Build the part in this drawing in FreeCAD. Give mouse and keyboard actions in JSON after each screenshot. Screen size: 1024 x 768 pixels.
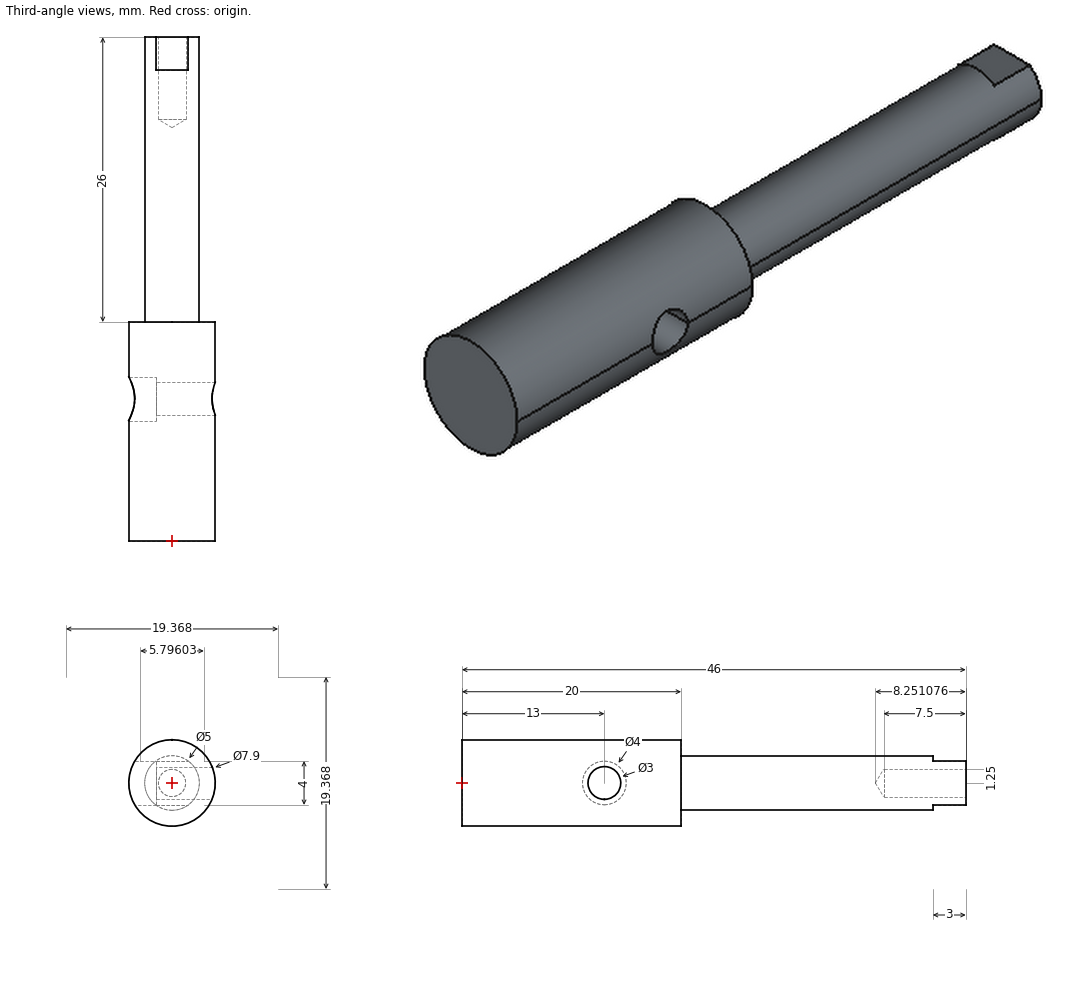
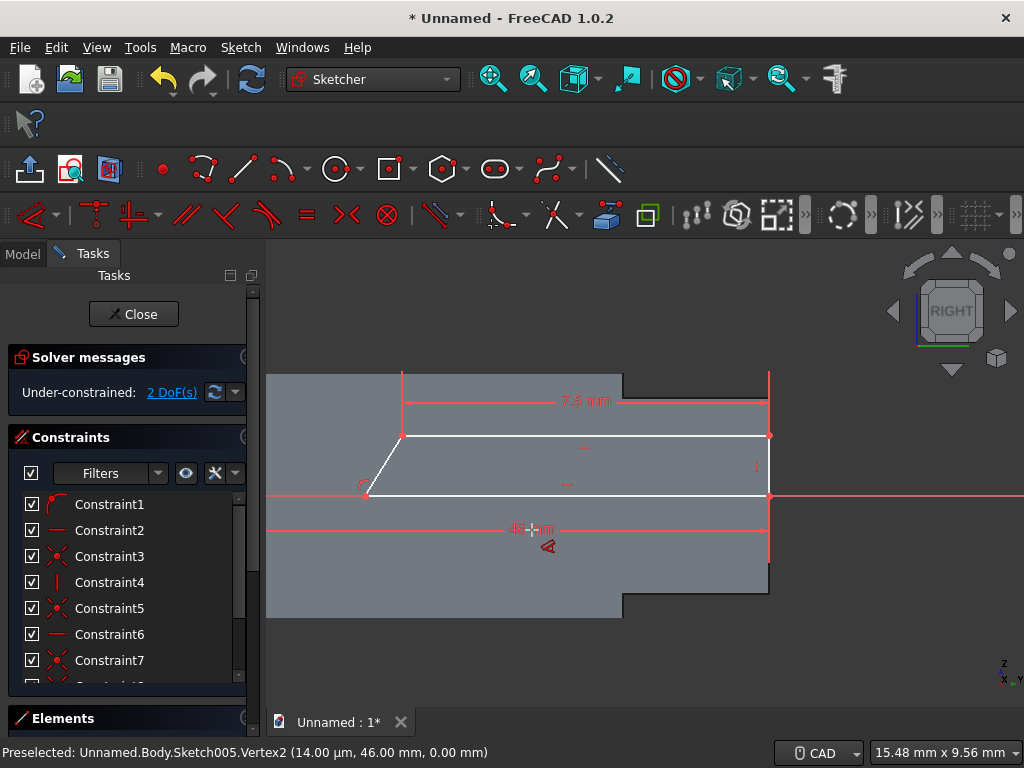
{"action": "left_click", "coordinate": [769, 478]}
{"action": "left_click", "coordinate": [803, 466]}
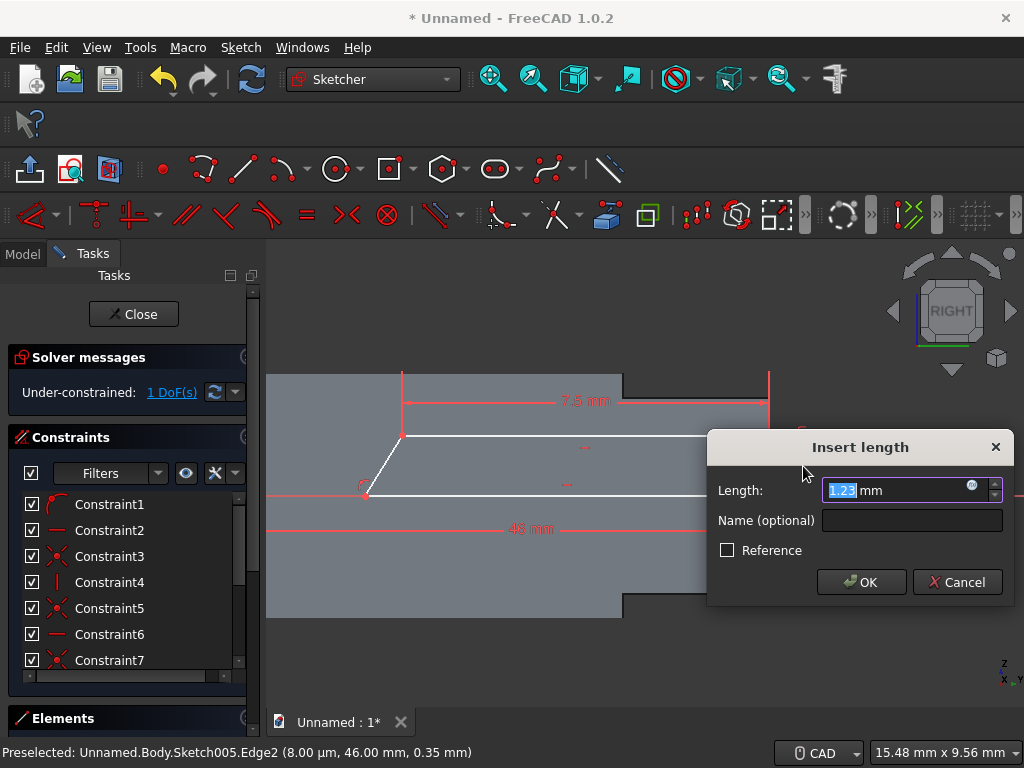
{"action": "type", "text": "1.25"}
{"action": "key", "text": "Return"}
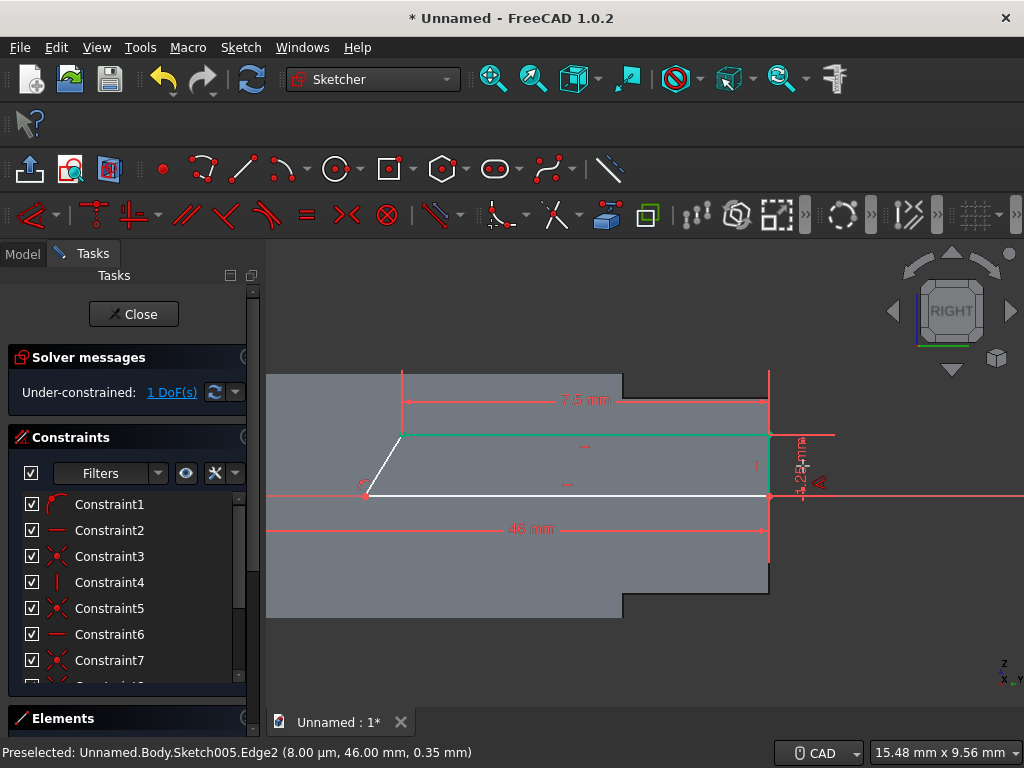
{"action": "left_click", "coordinate": [486, 496]}
{"action": "left_click", "coordinate": [660, 530]}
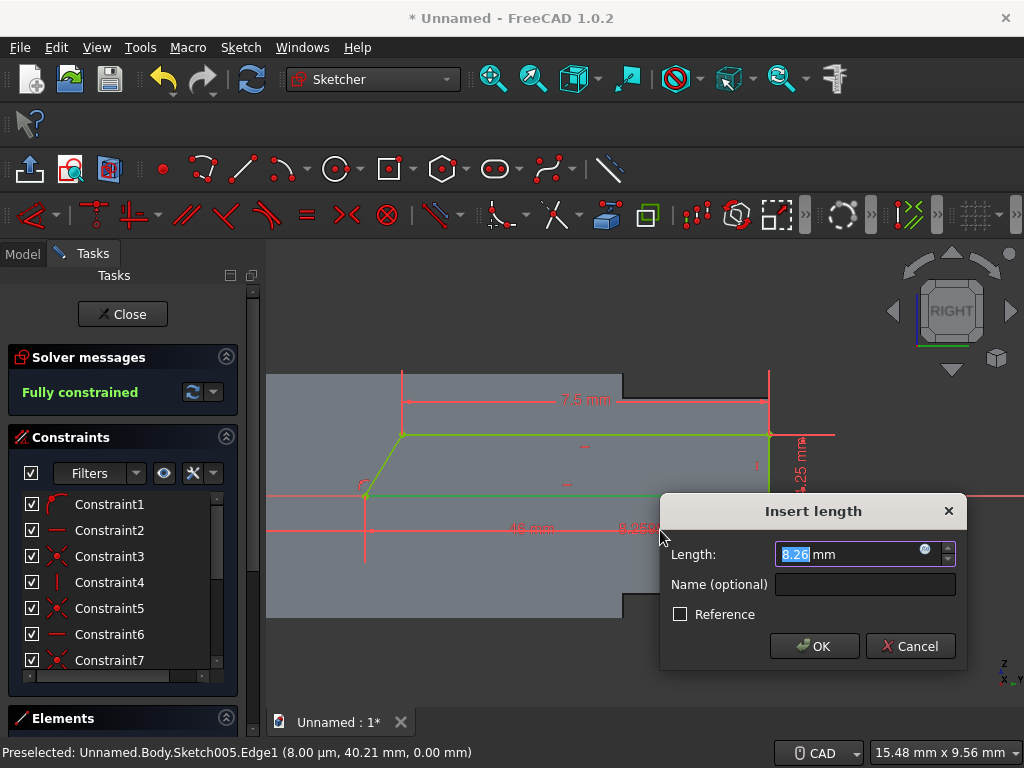
{"action": "type", "text": "8.251076"}
{"action": "key", "text": "Return"}
{"action": "key", "text": "Escape"}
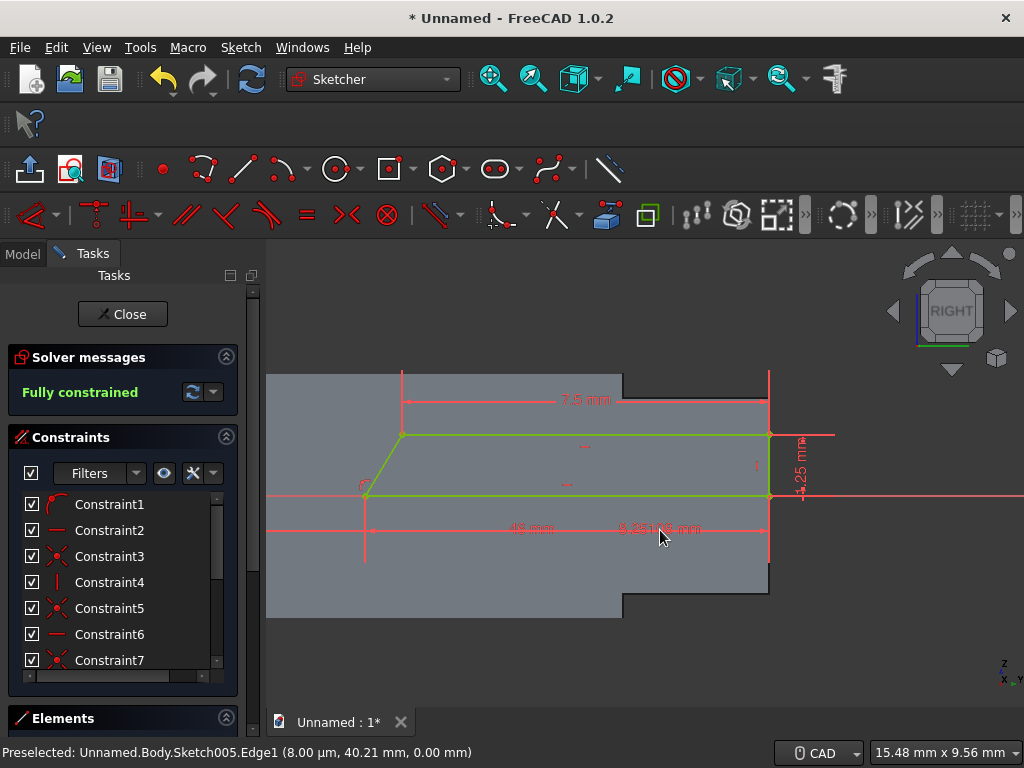
{"action": "left_click", "coordinate": [123, 314]}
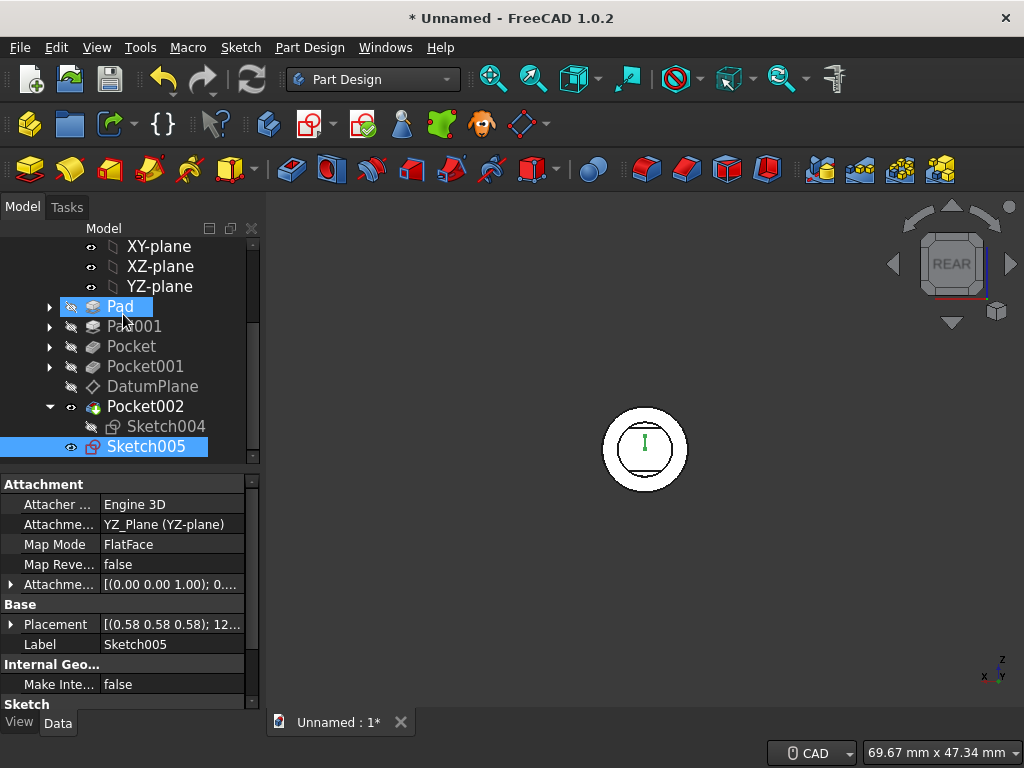
{"action": "left_click", "coordinate": [372, 170]}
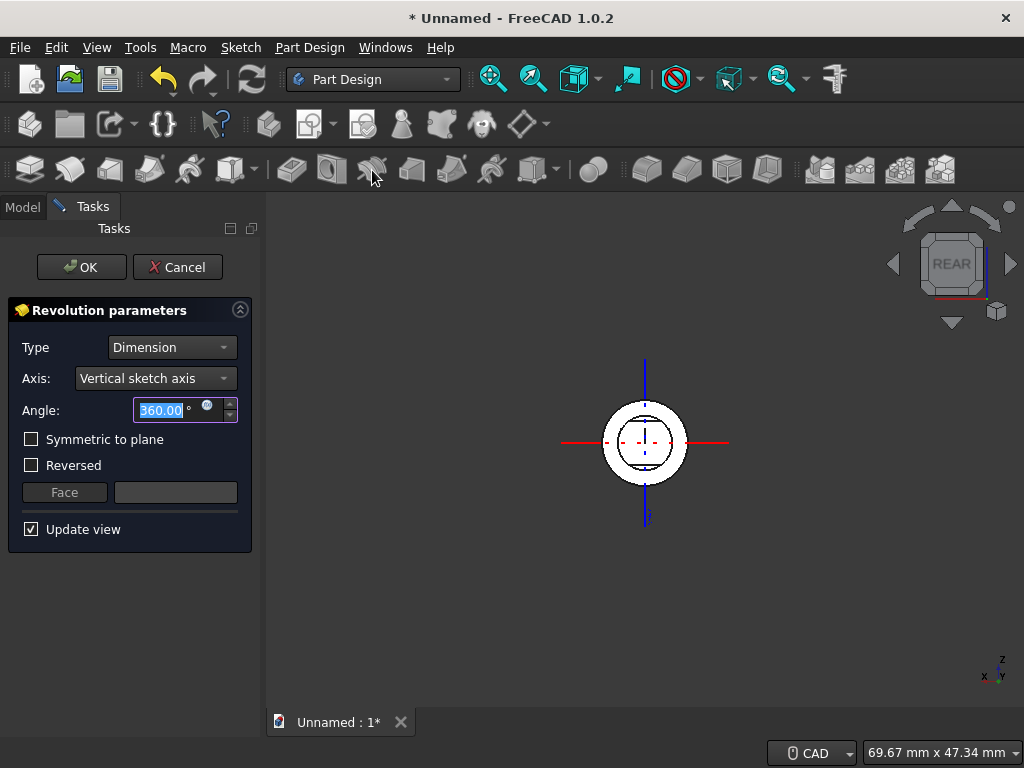
{"action": "left_click", "coordinate": [156, 378]}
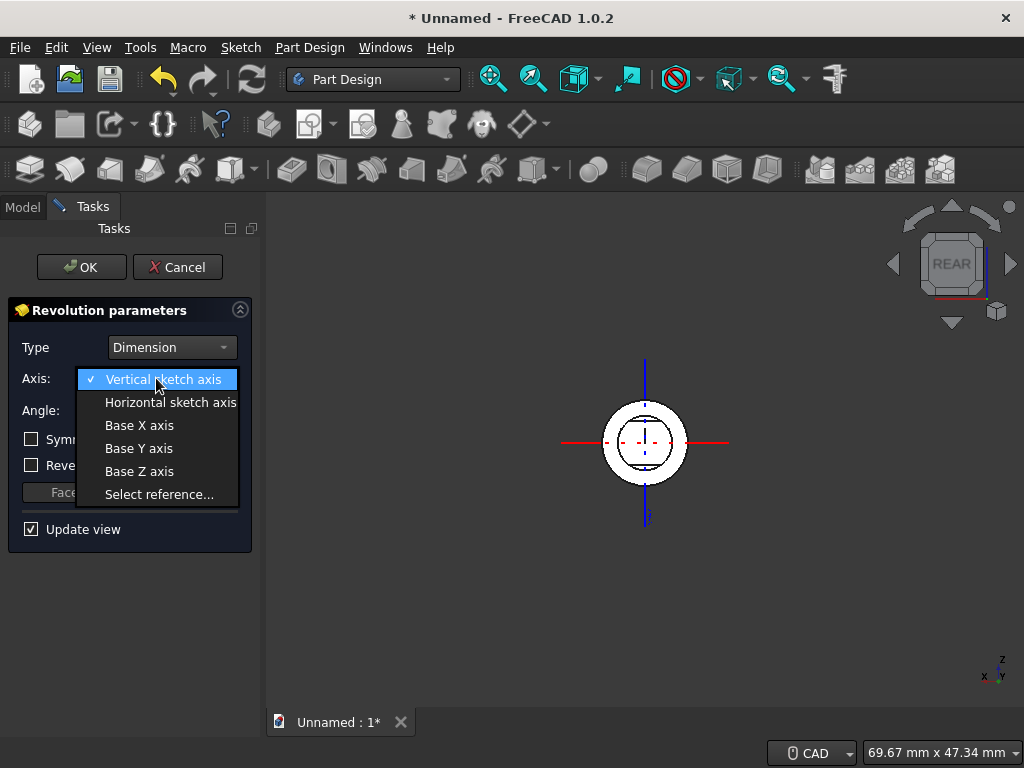
{"action": "left_click", "coordinate": [156, 402]}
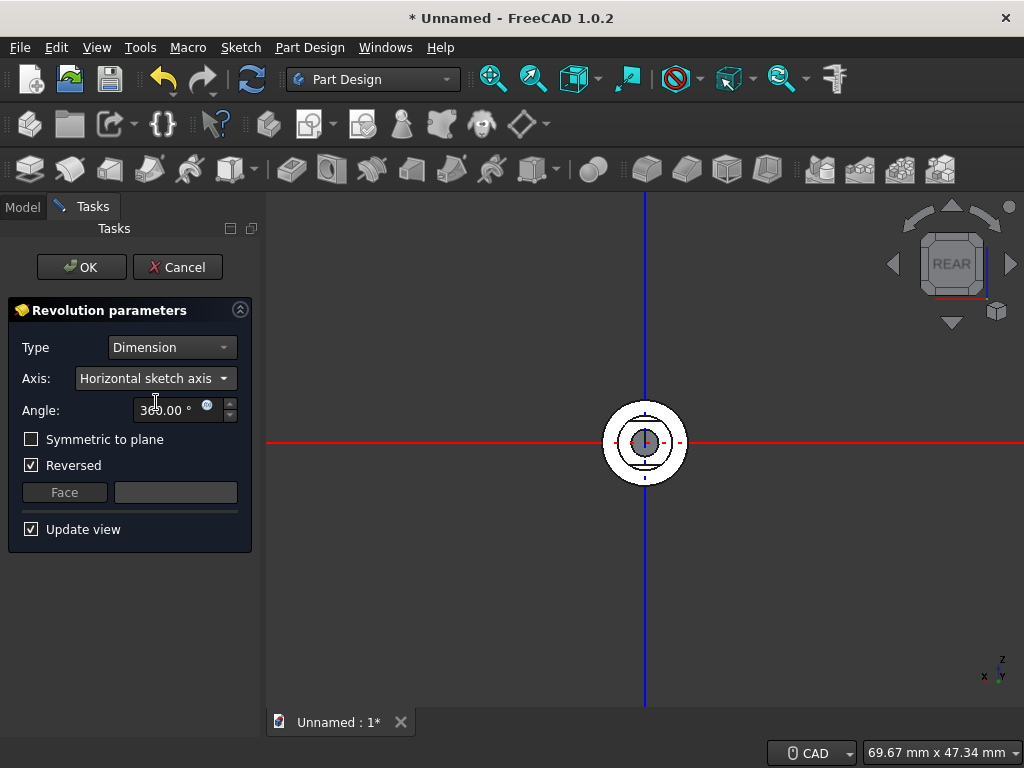
{"action": "left_click", "coordinate": [82, 267]}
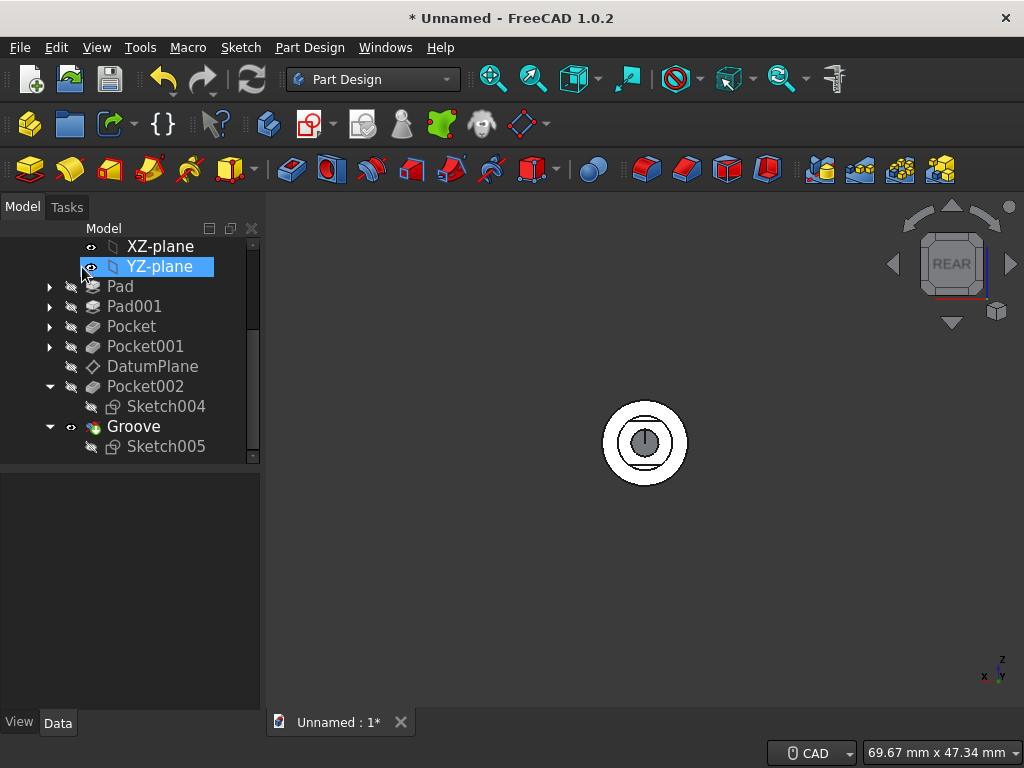
{"action": "key", "text": "0"}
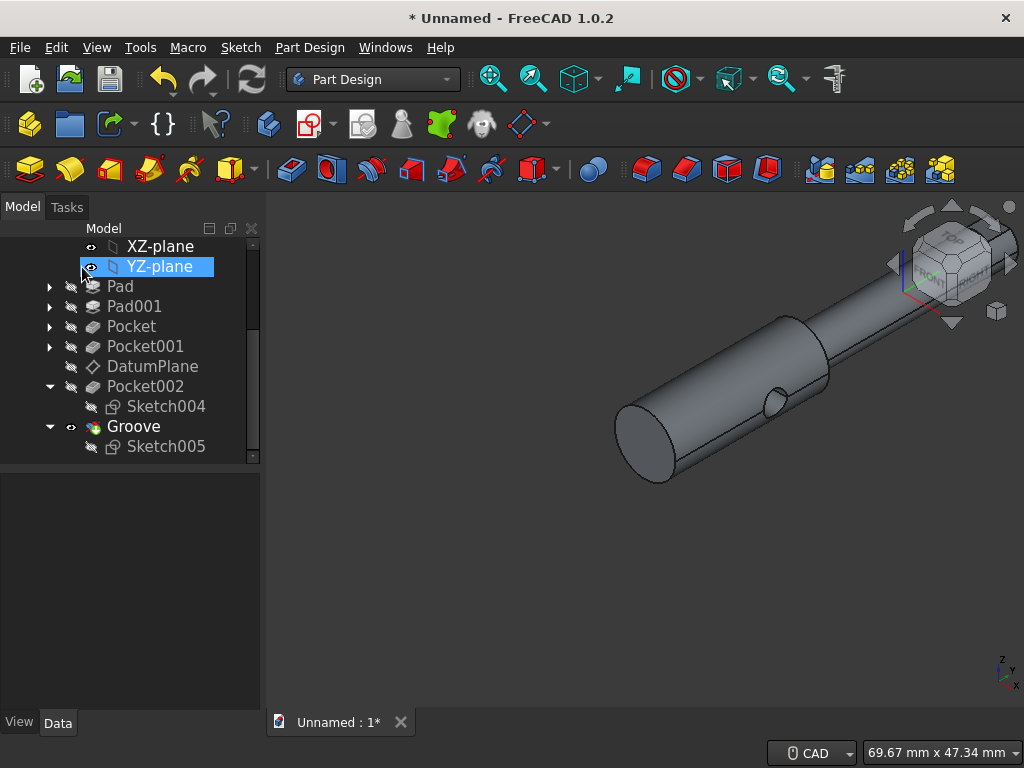
{"action": "left_click", "coordinate": [494, 80]}